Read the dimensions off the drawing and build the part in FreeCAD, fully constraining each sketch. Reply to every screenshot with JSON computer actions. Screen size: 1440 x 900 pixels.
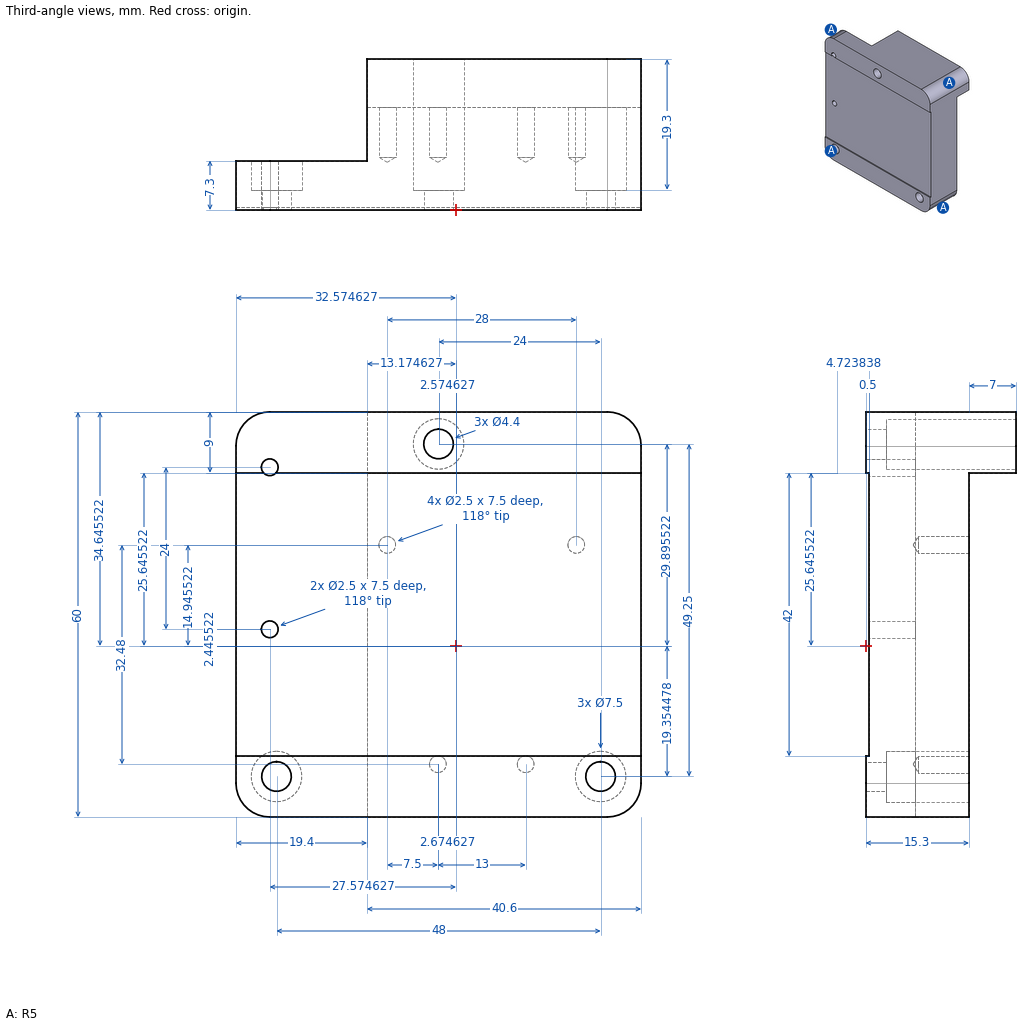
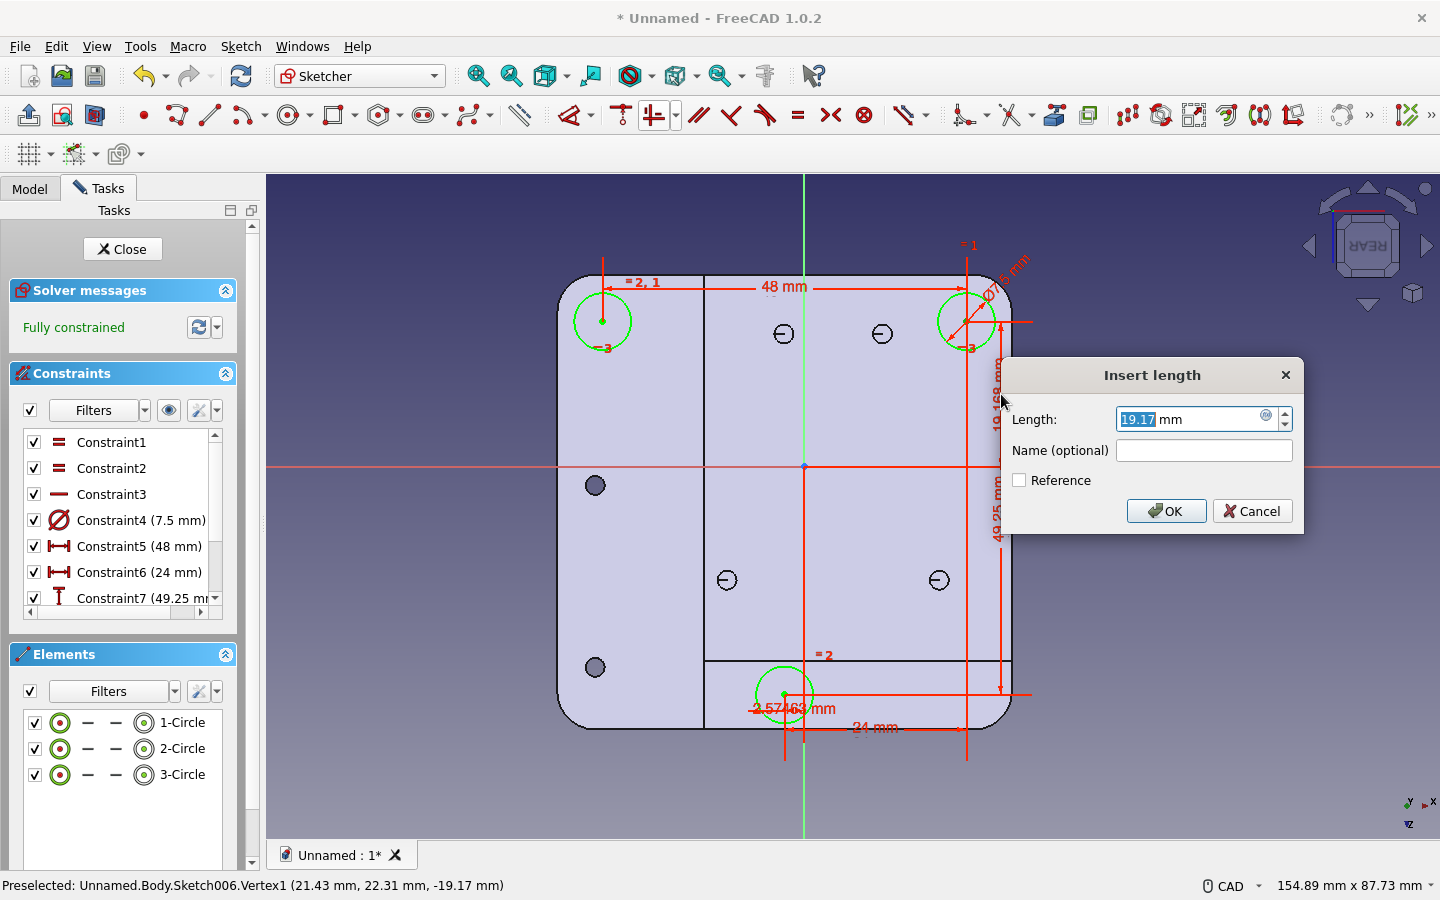
{"action": "type", "text": "19.354478"}
{"action": "key", "text": "Return"}
{"action": "key", "text": "Escape"}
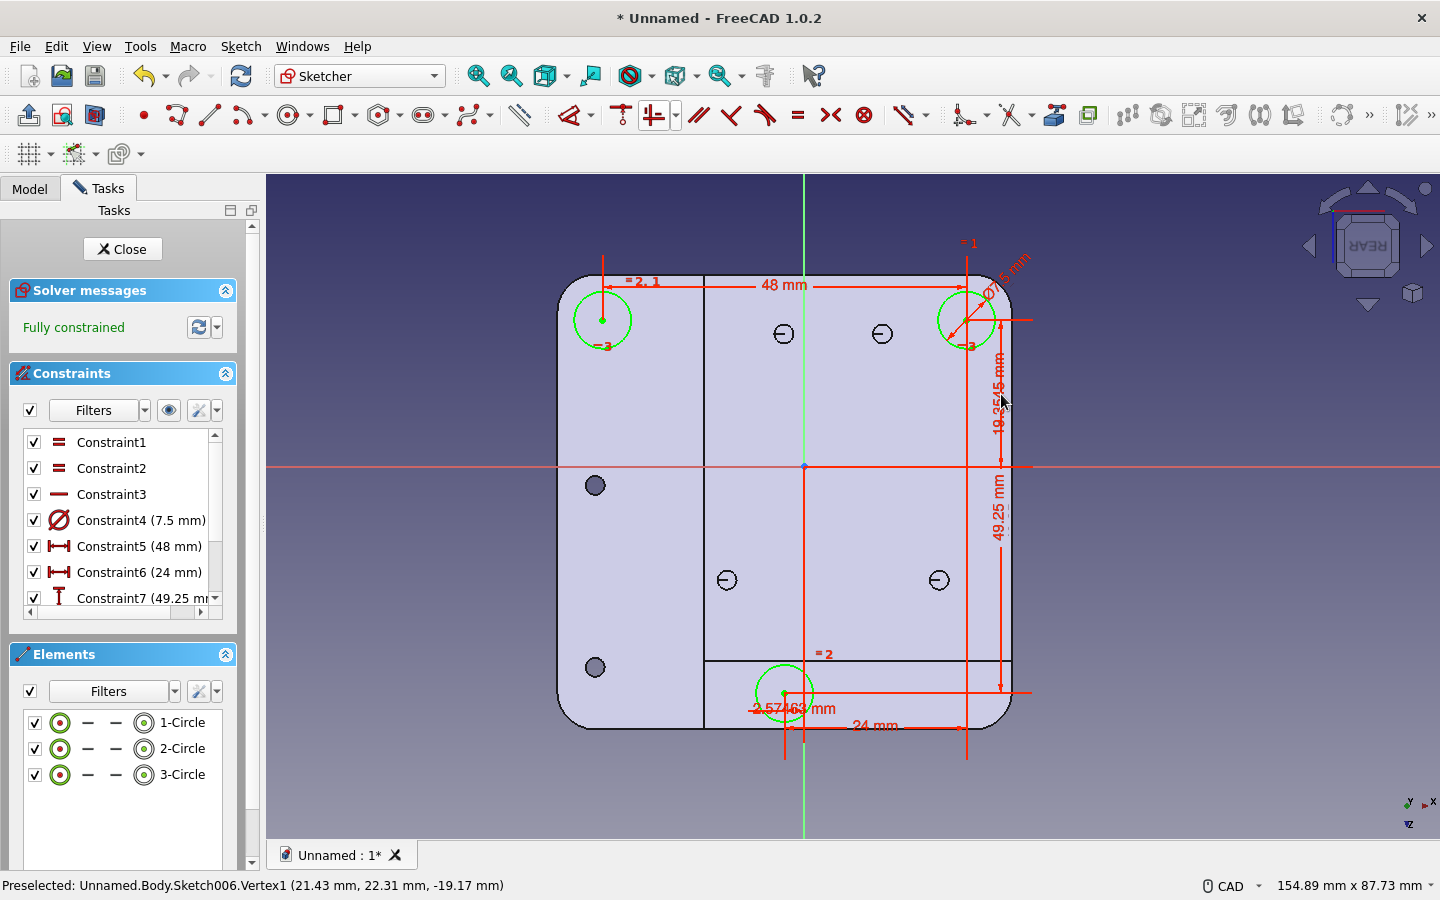
{"action": "left_click", "coordinate": [123, 249]}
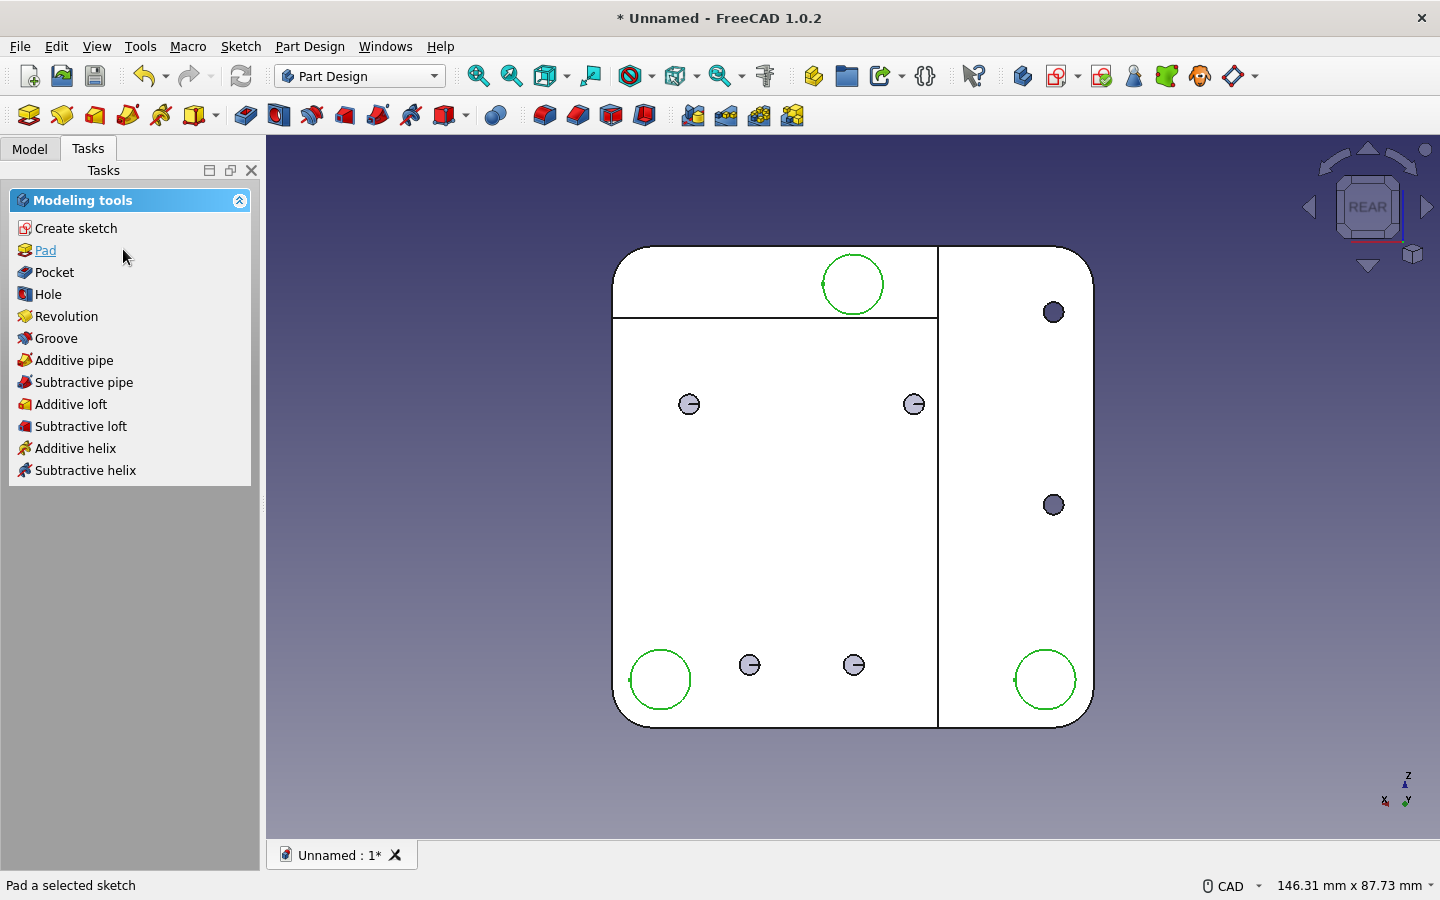
{"action": "left_click", "coordinate": [246, 116]}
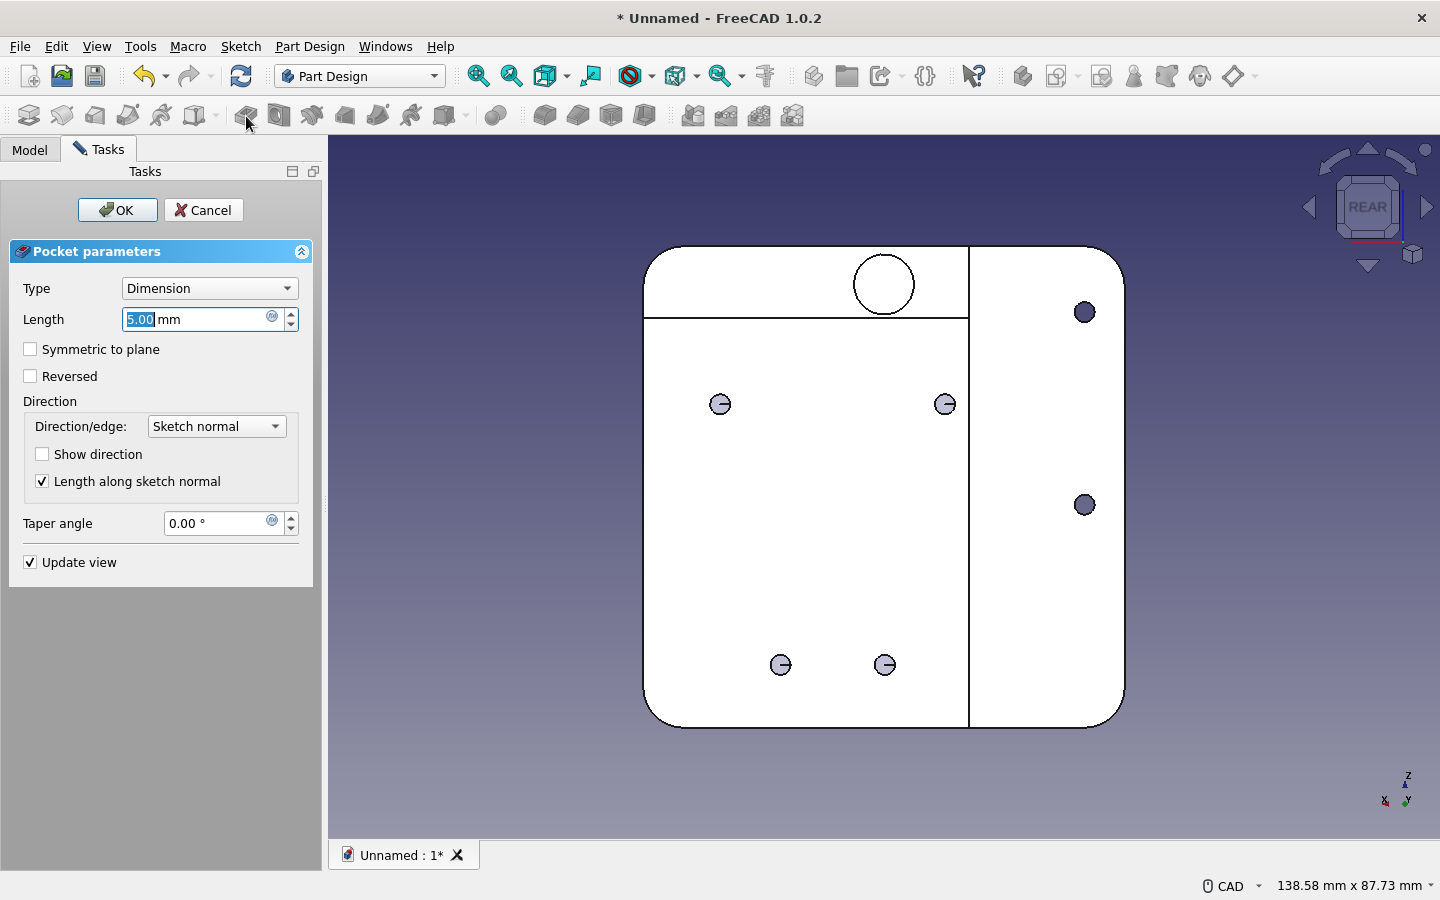
{"action": "type", "text": "19.3"}
{"action": "key", "text": "Tab"}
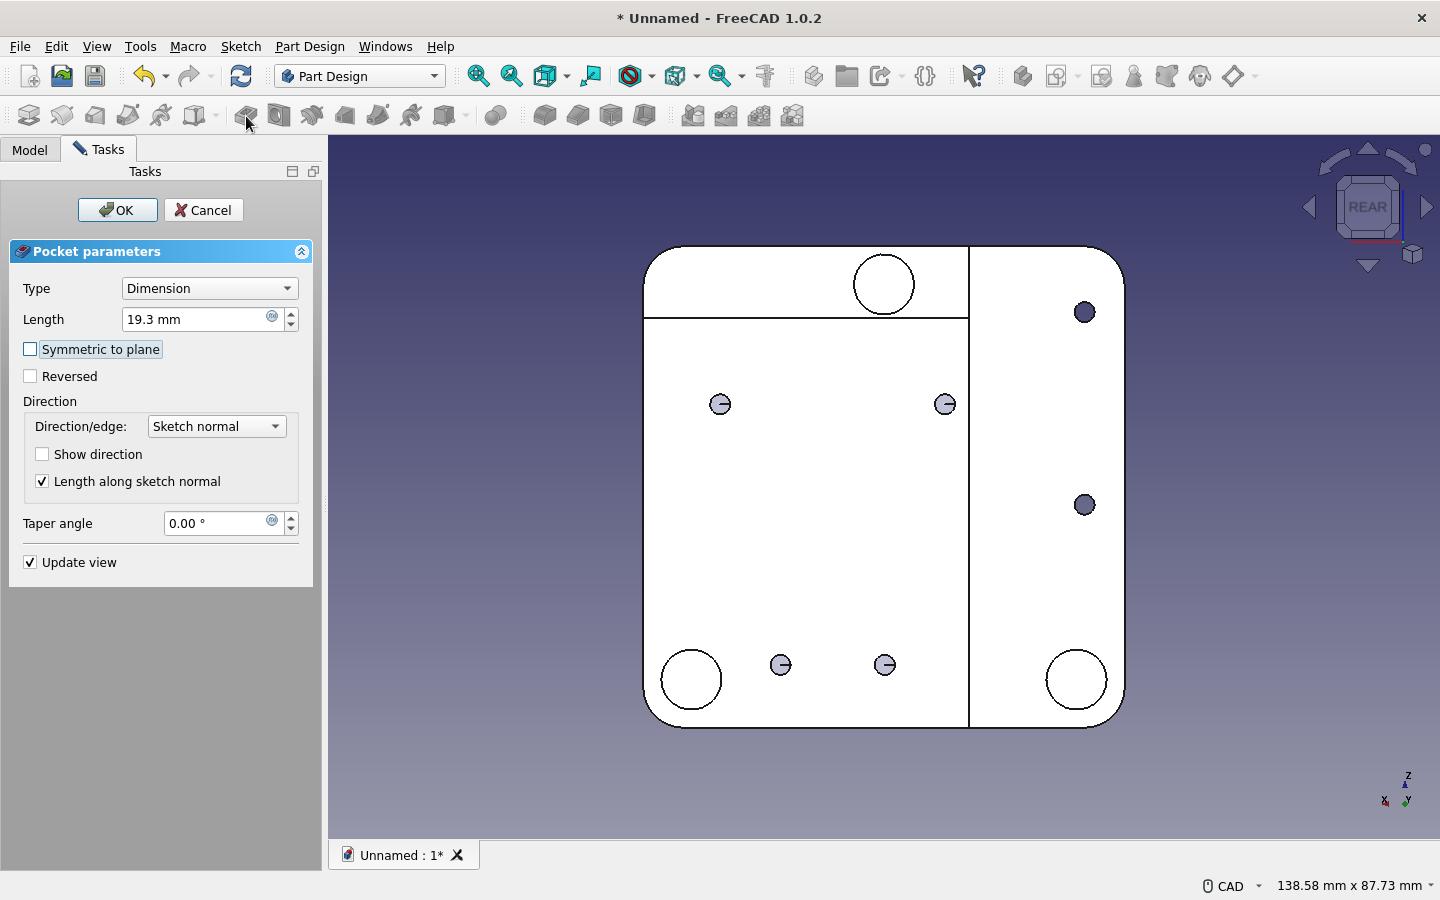
{"action": "left_click", "coordinate": [118, 210]}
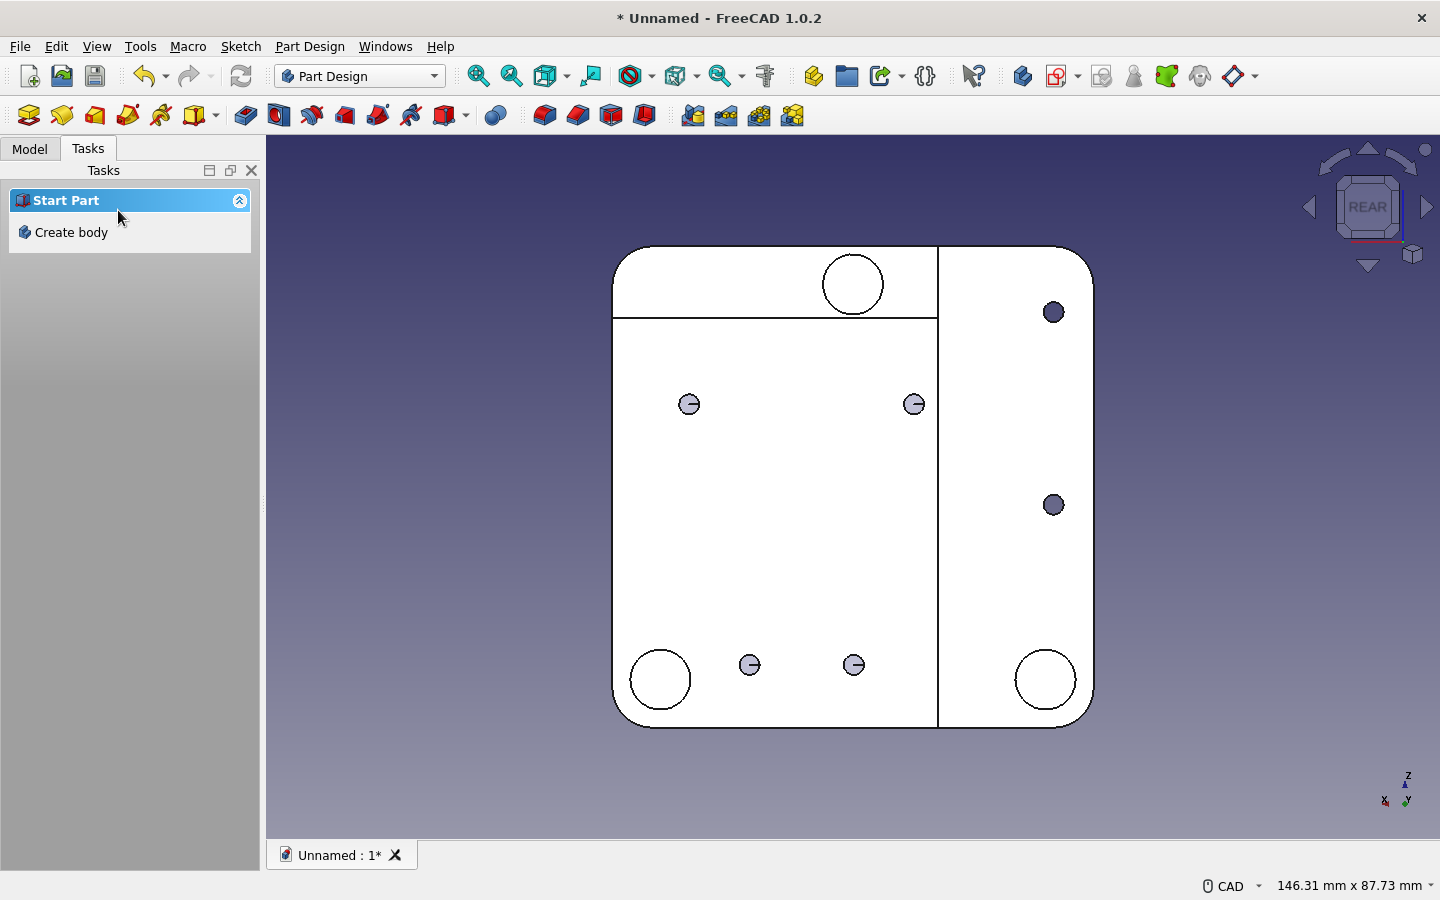
{"action": "left_click", "coordinate": [660, 679]}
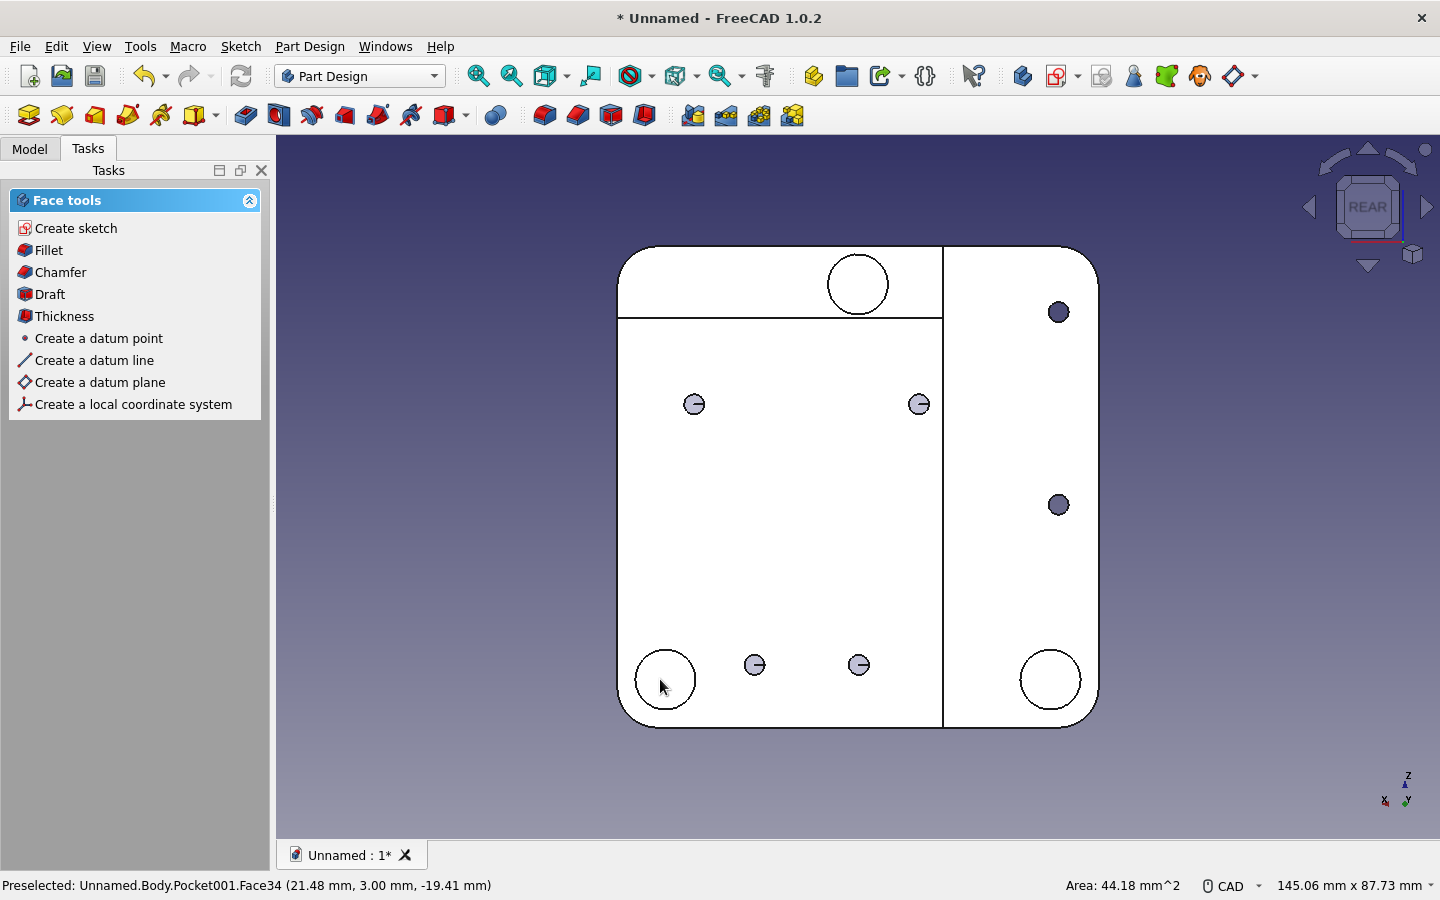
{"action": "left_click", "coordinate": [1056, 76]}